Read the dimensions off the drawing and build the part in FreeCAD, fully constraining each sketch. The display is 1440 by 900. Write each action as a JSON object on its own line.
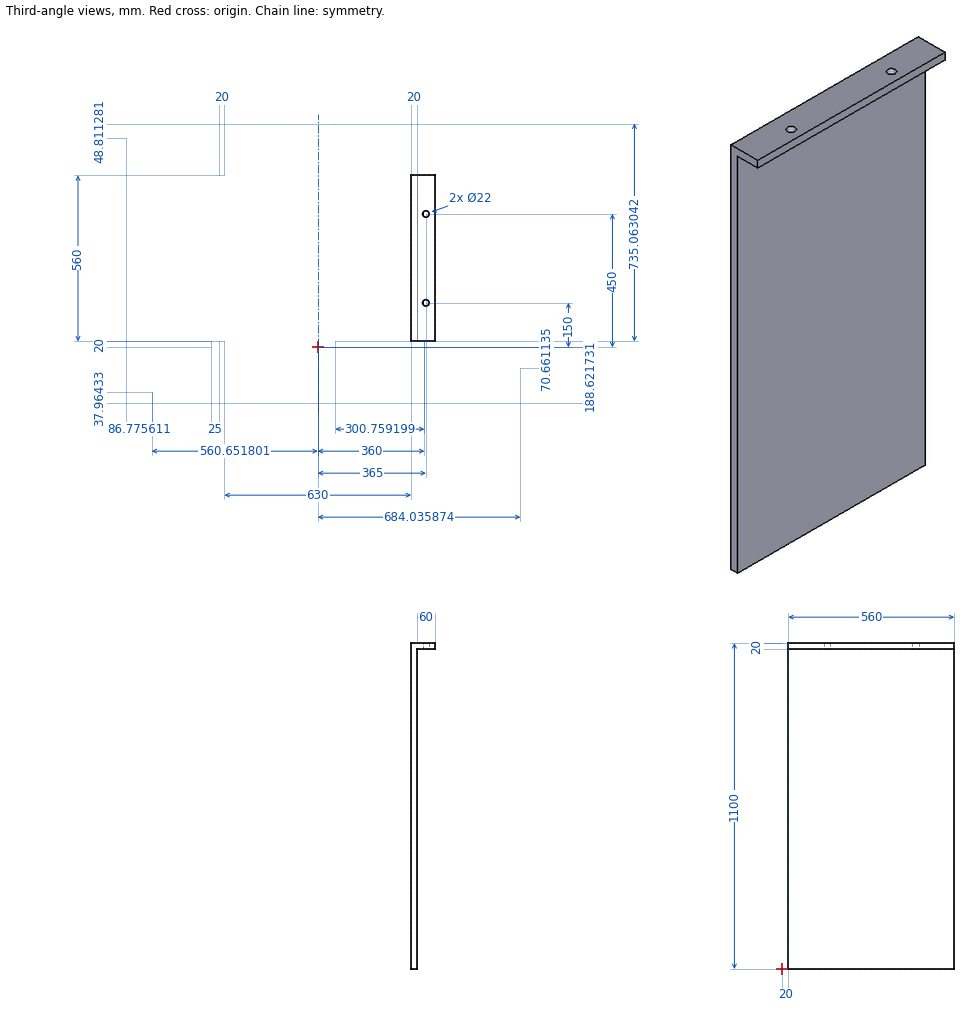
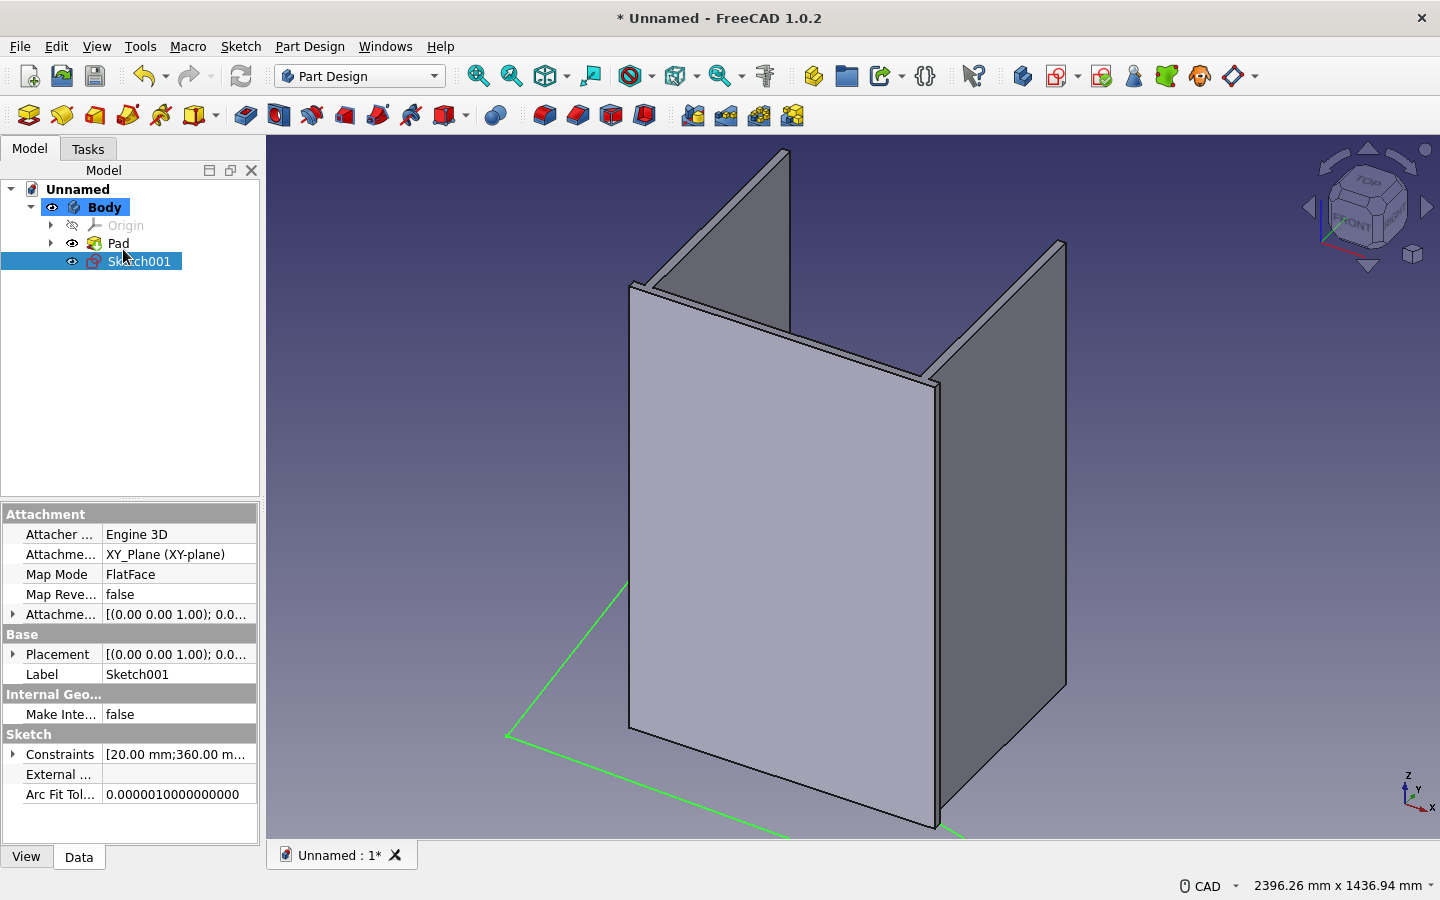
{"action": "left_click", "coordinate": [246, 116]}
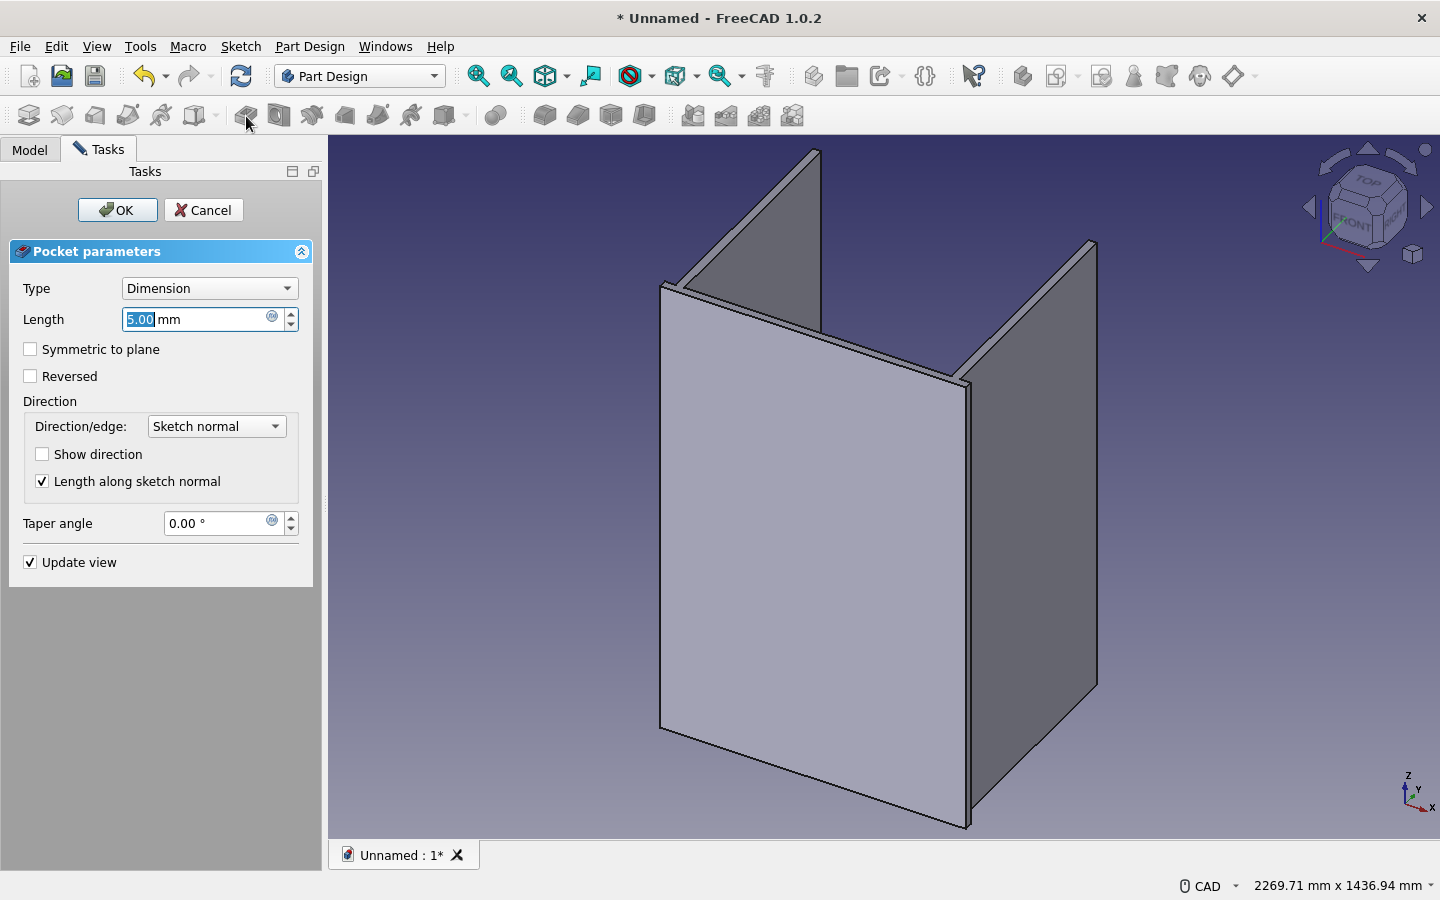
{"action": "left_click", "coordinate": [210, 288]}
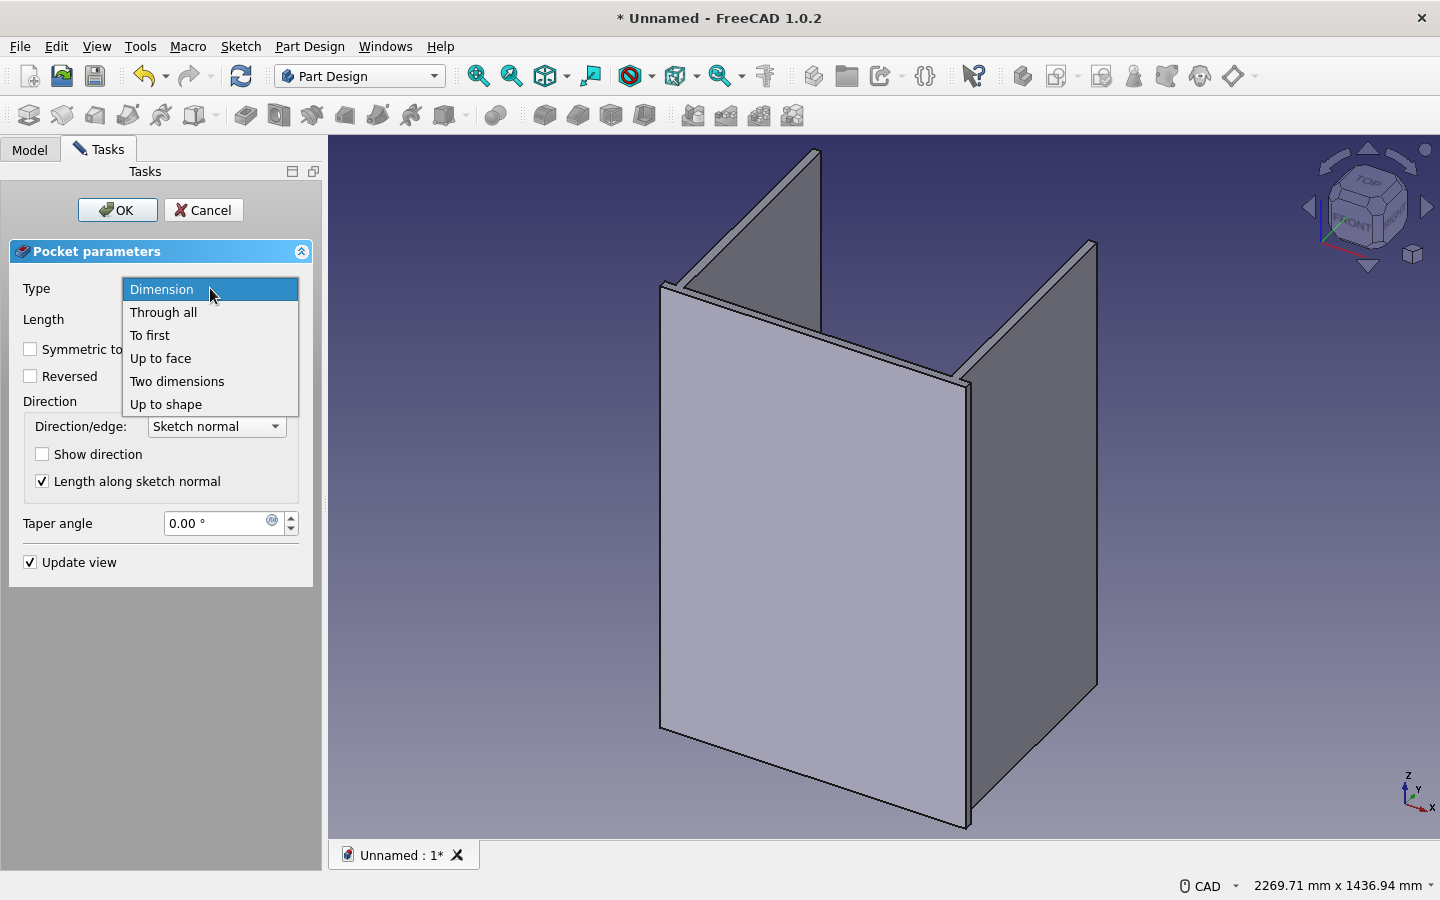
{"action": "left_click", "coordinate": [208, 312]}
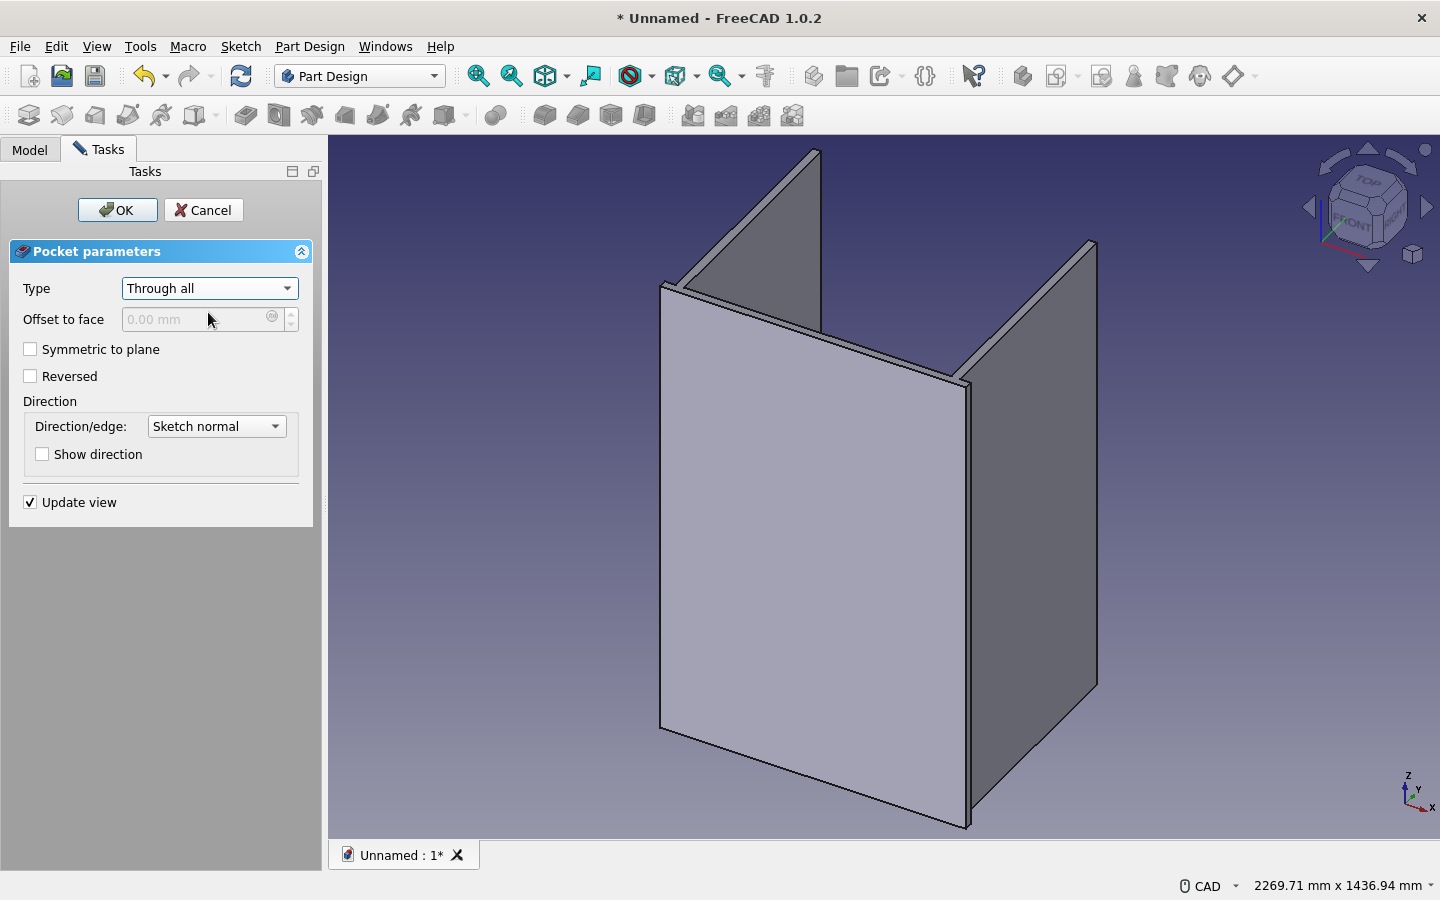
{"action": "left_click", "coordinate": [31, 376]}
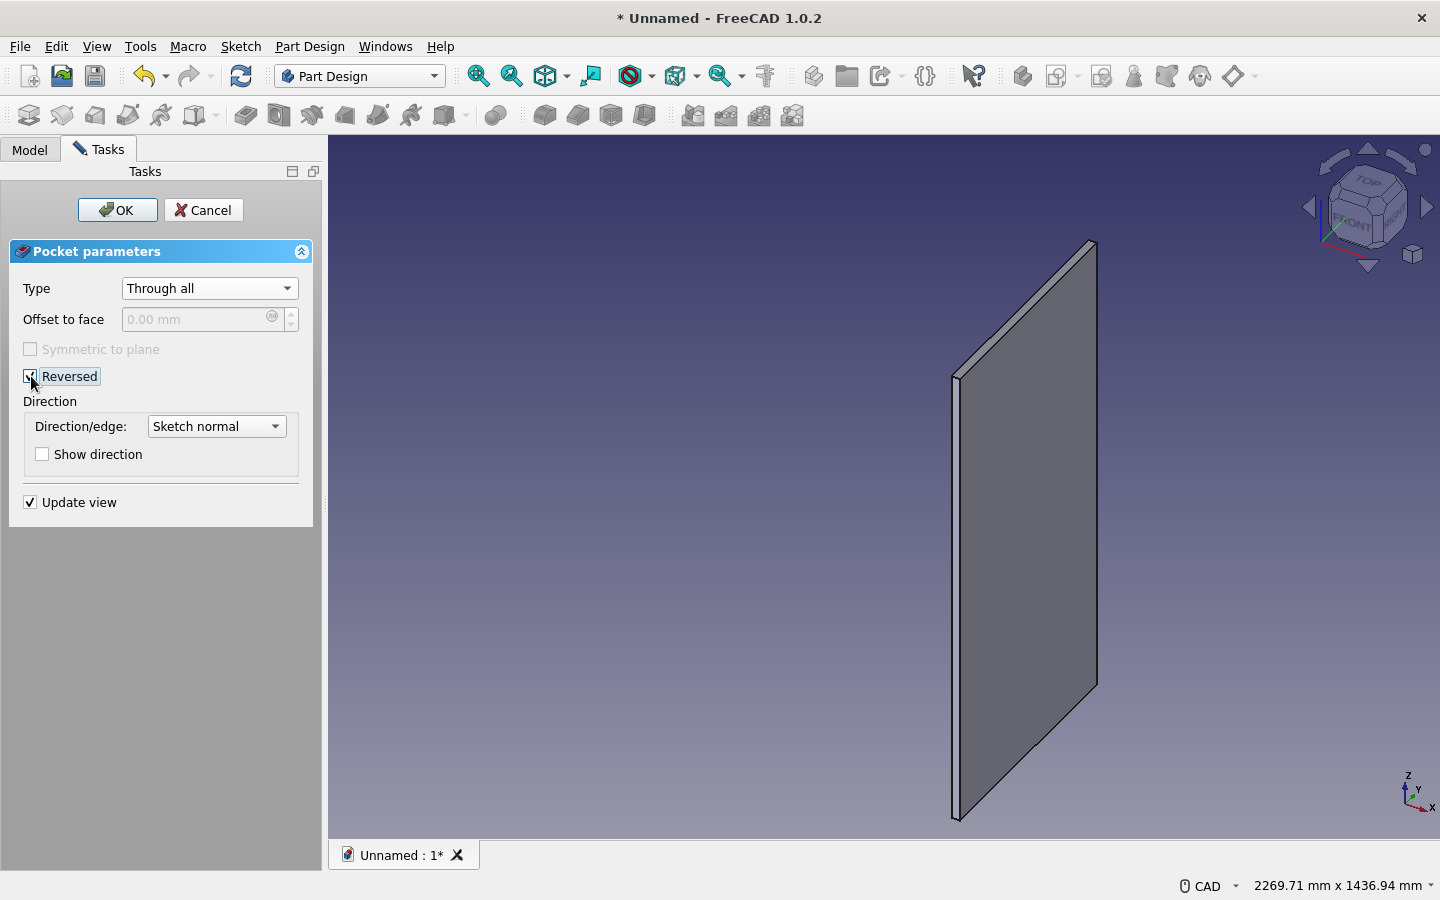
{"action": "left_click", "coordinate": [118, 210]}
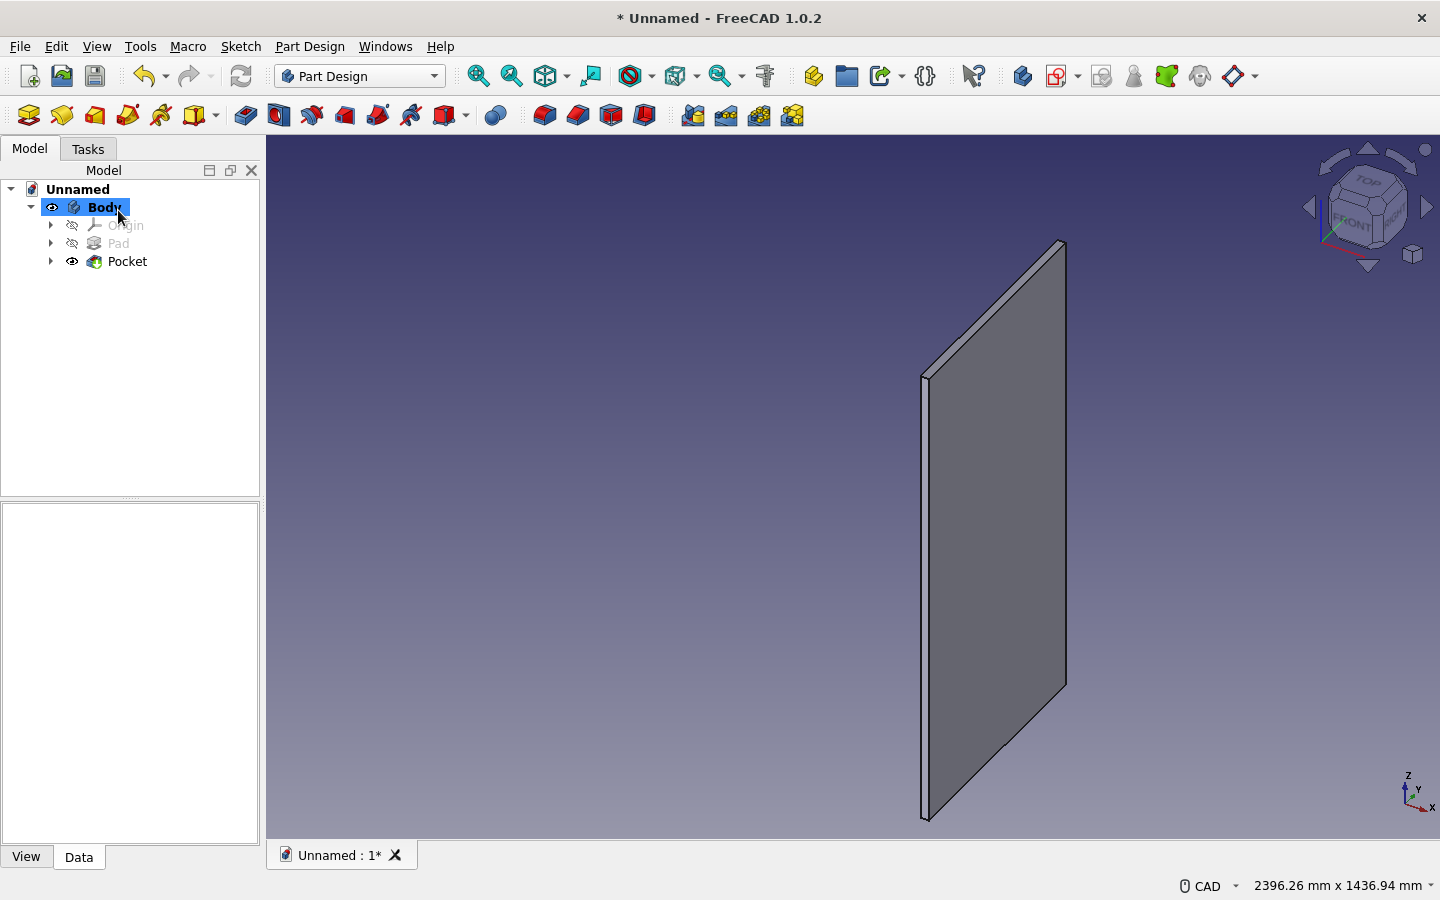
{"action": "left_click", "coordinate": [998, 468]}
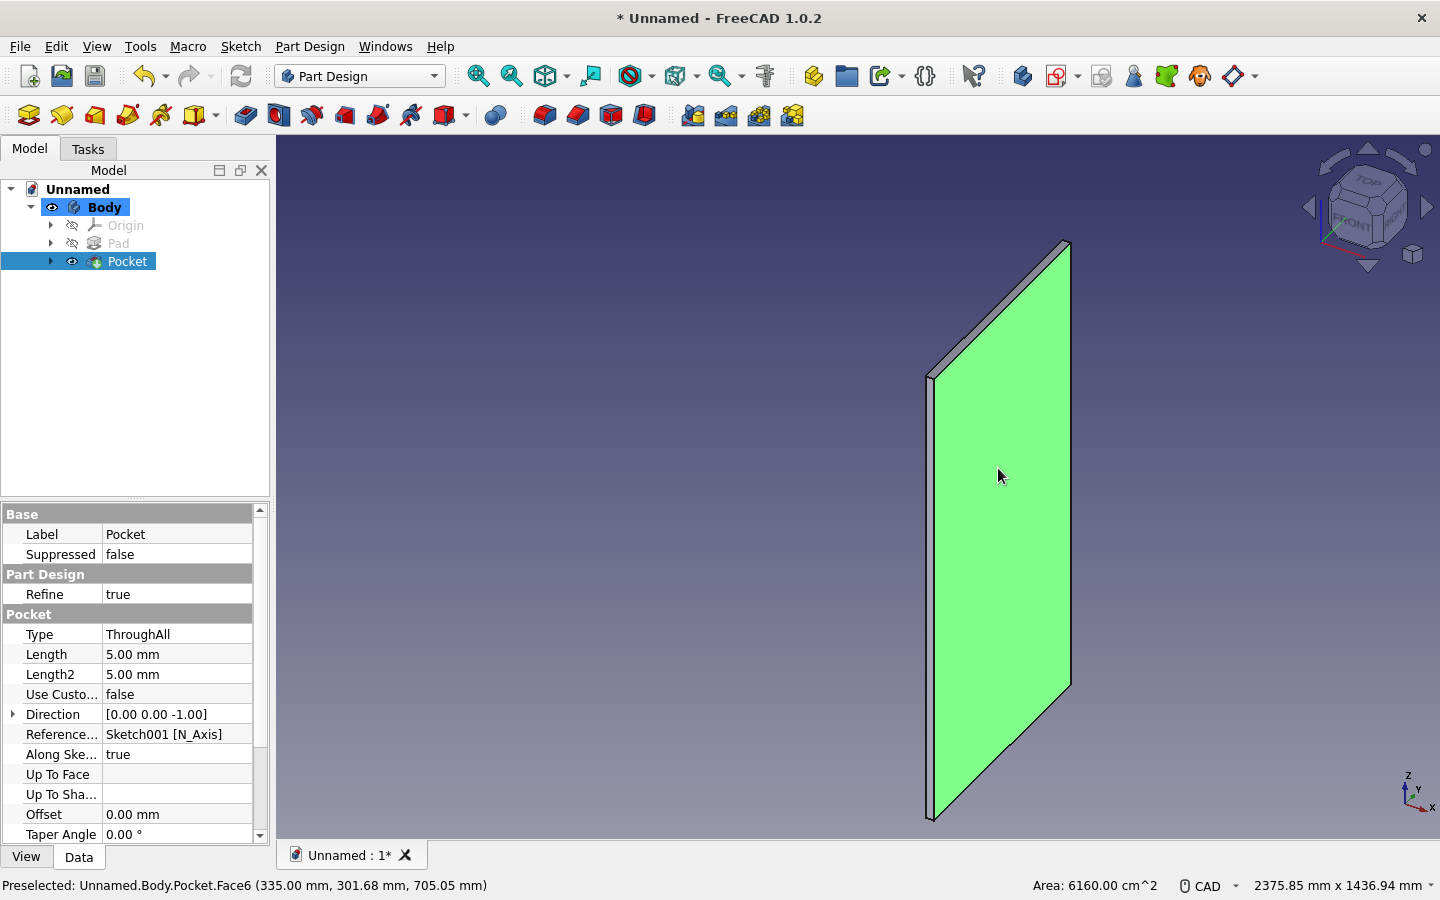
{"action": "left_click", "coordinate": [1056, 76]}